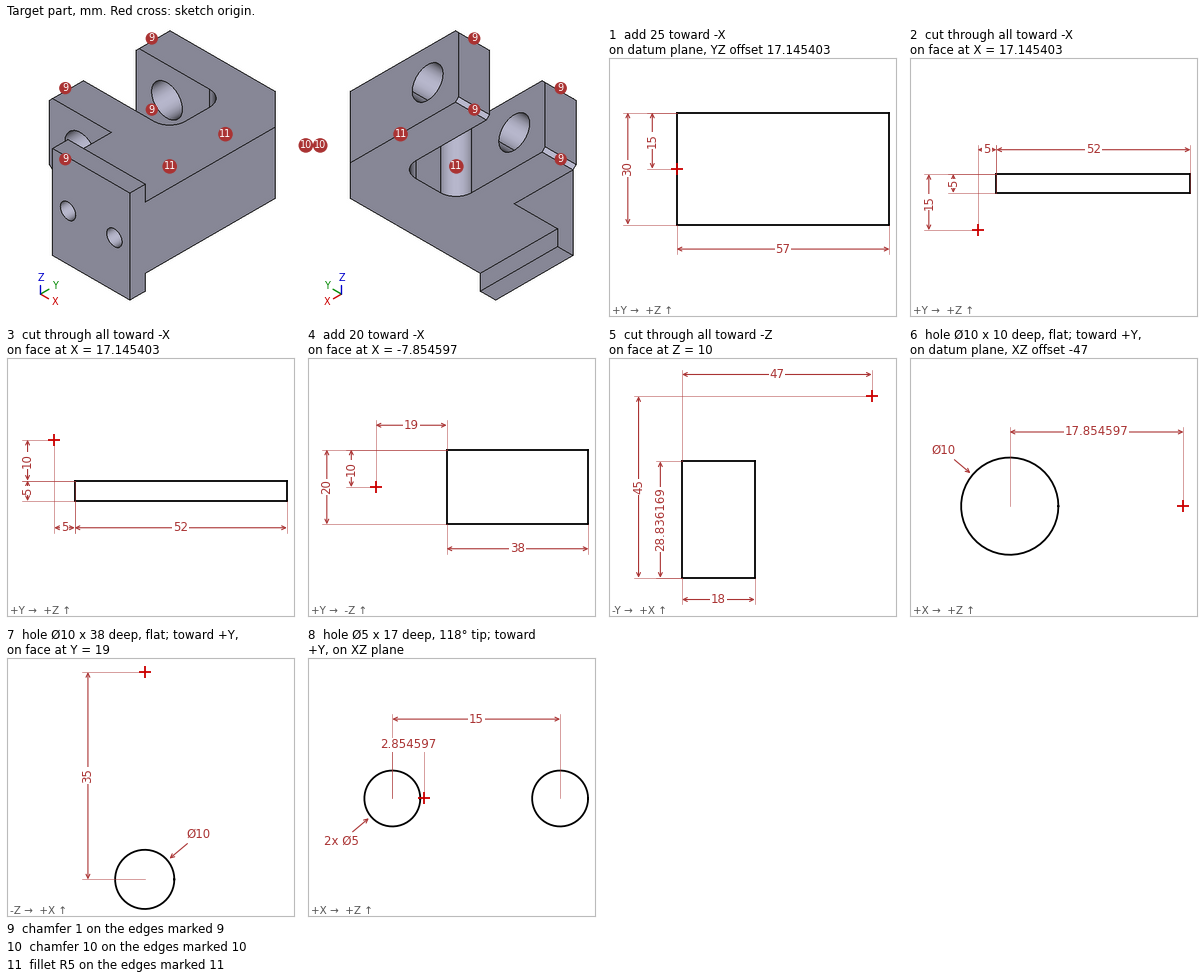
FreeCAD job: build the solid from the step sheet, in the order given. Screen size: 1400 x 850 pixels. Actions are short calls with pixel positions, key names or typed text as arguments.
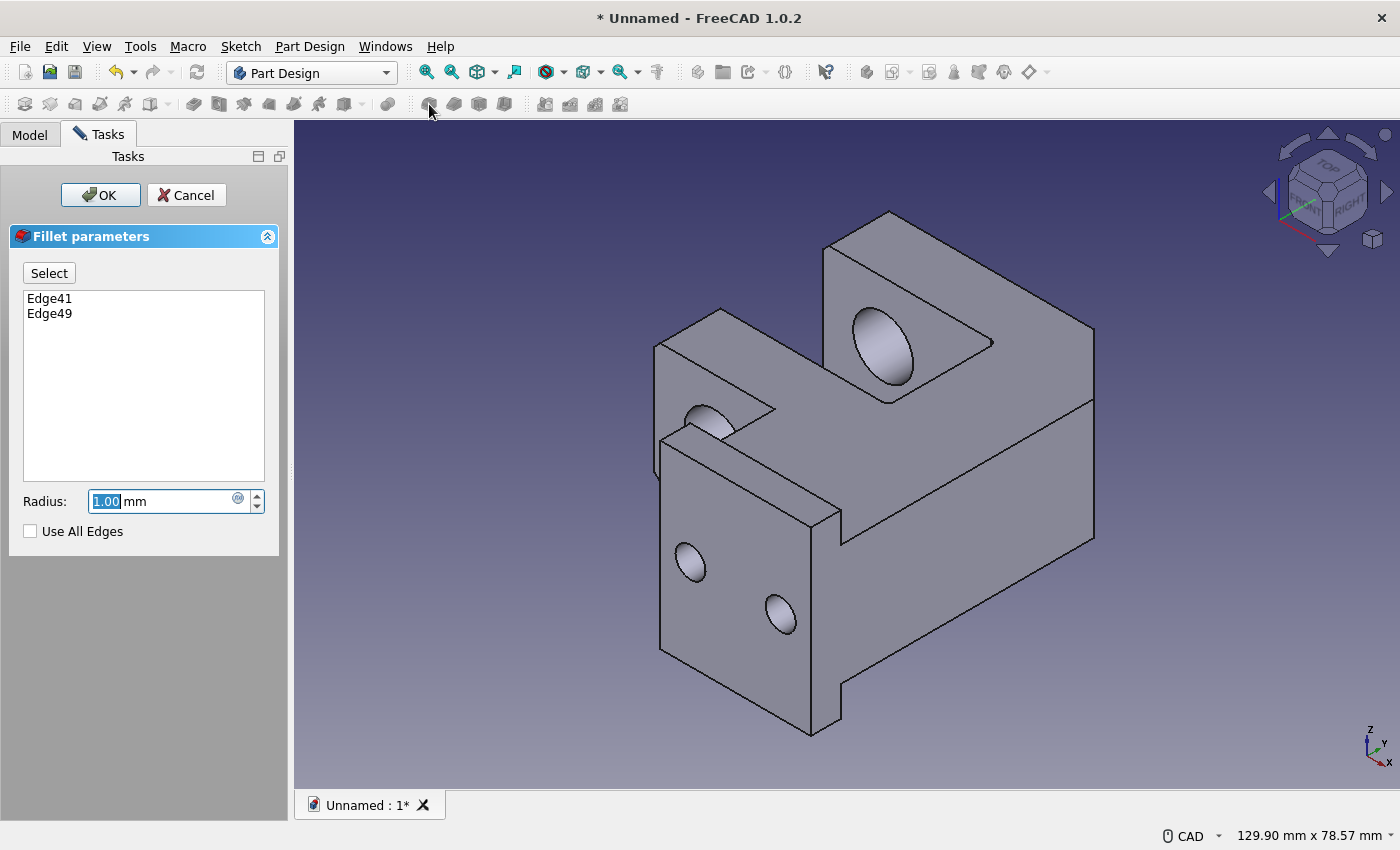
text(5)
key(Tab)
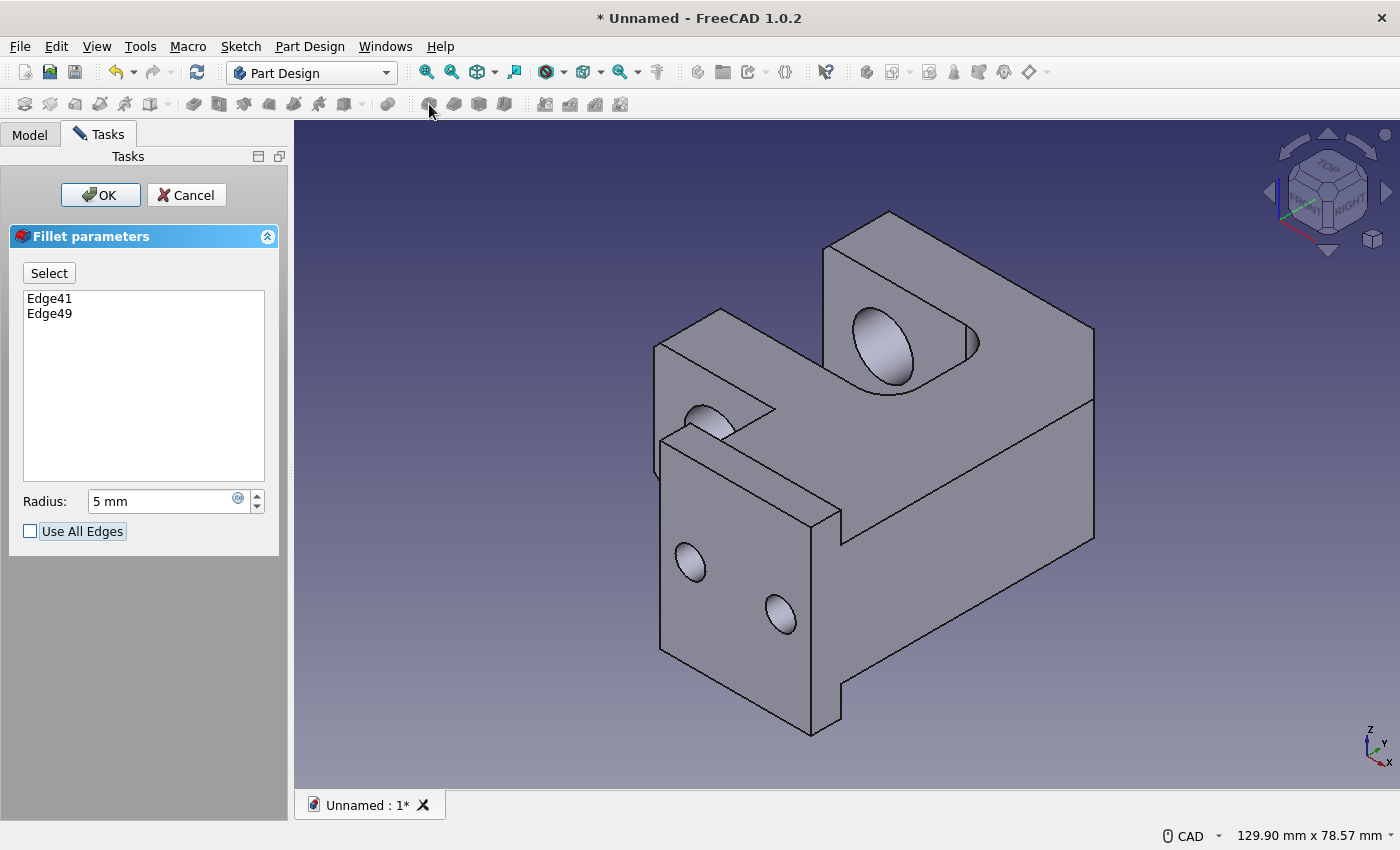
click(101, 195)